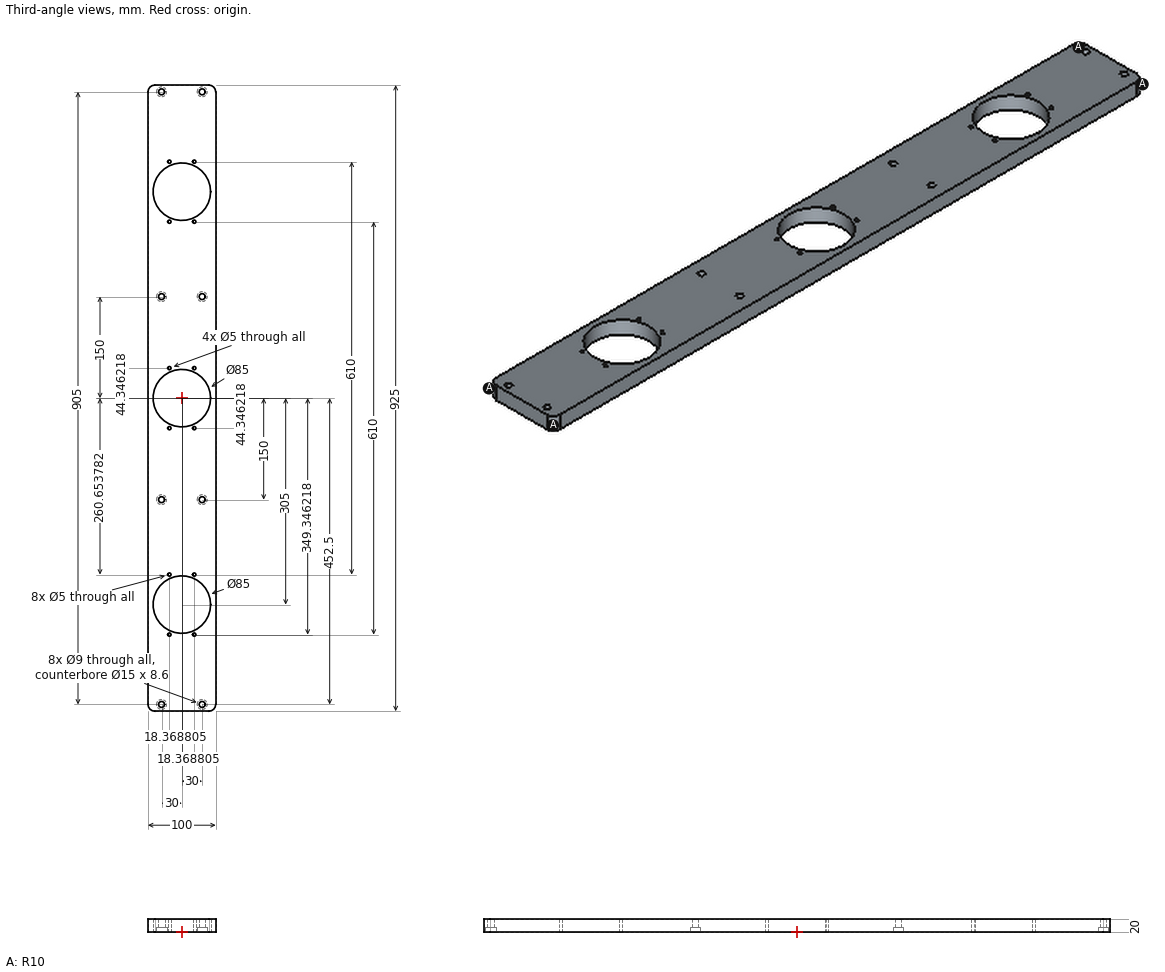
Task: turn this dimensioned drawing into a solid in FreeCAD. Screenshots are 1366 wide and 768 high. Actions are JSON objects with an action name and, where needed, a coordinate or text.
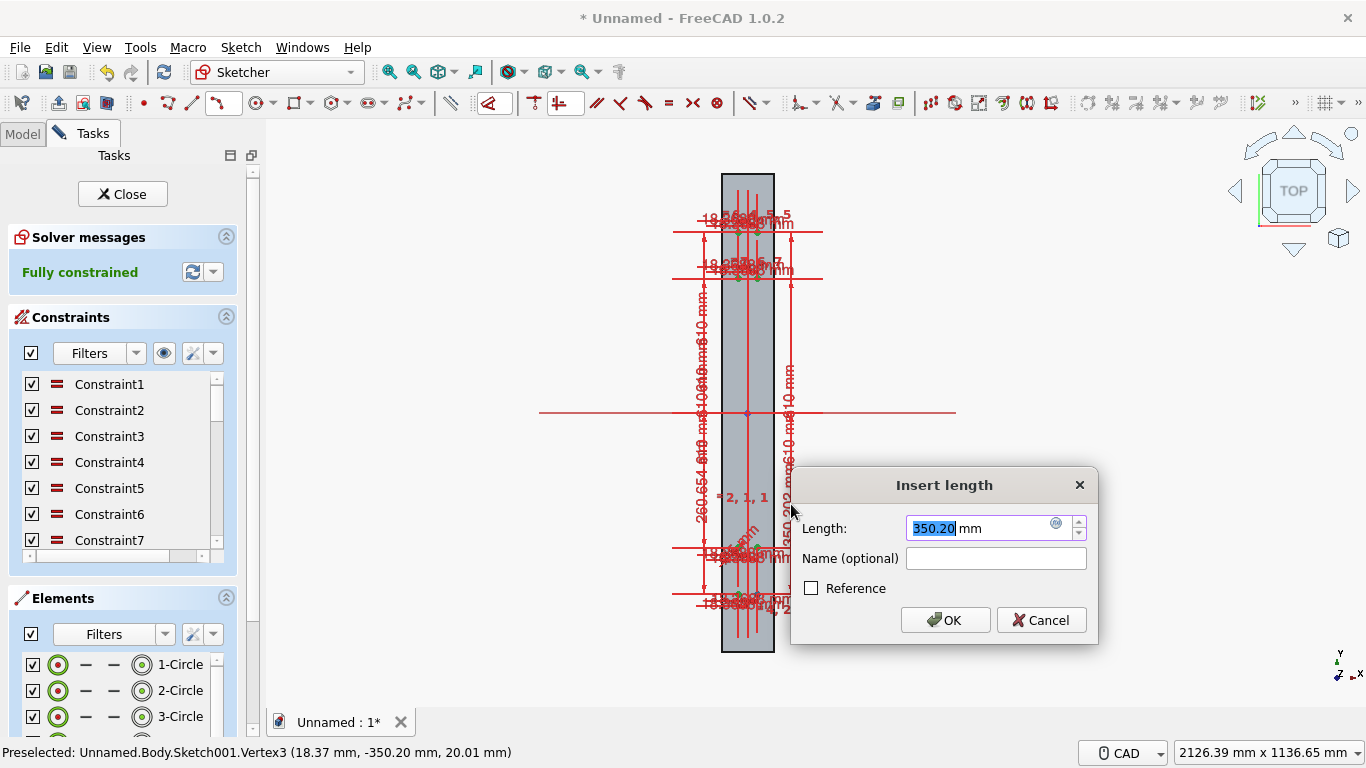
{"action": "type", "text": "349.346218"}
{"action": "key", "text": "Return"}
{"action": "key", "text": "Escape"}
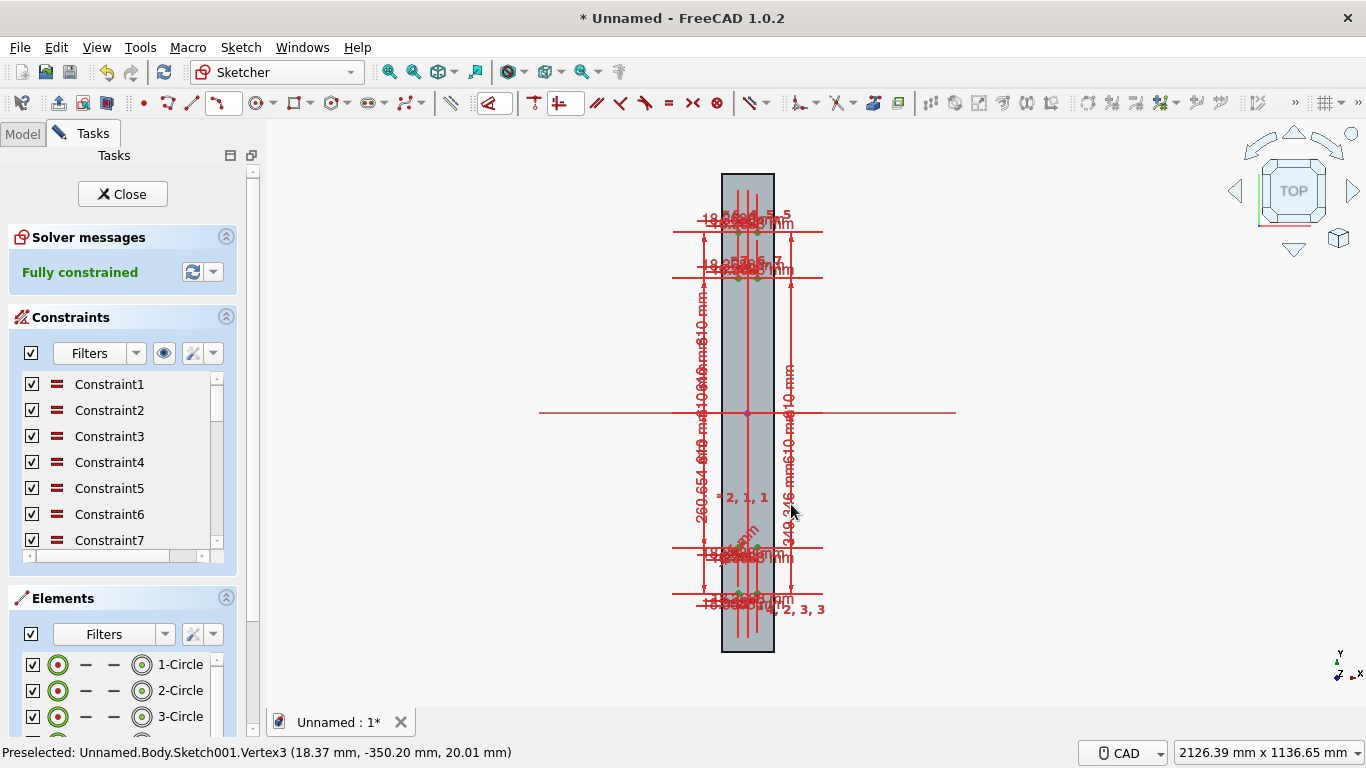
{"action": "left_click", "coordinate": [123, 194]}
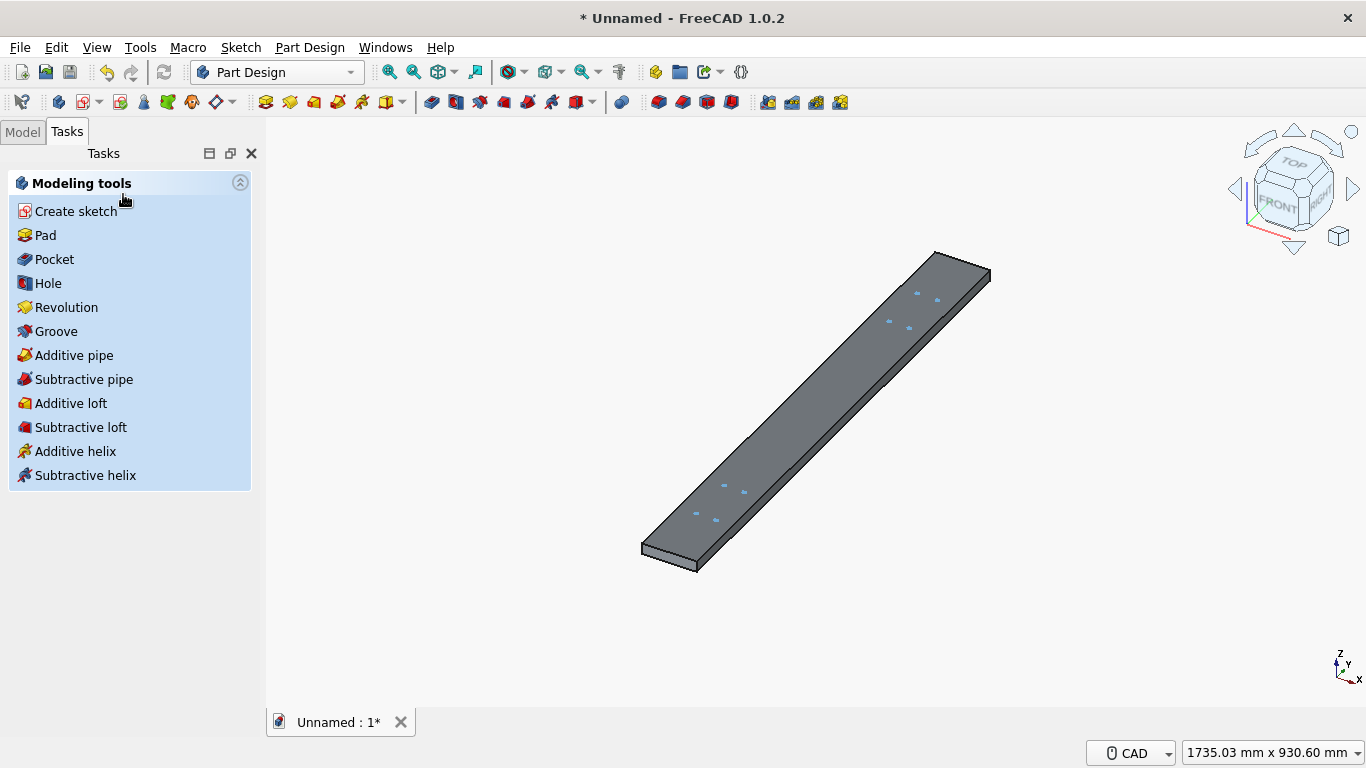
{"action": "left_click", "coordinate": [456, 102]}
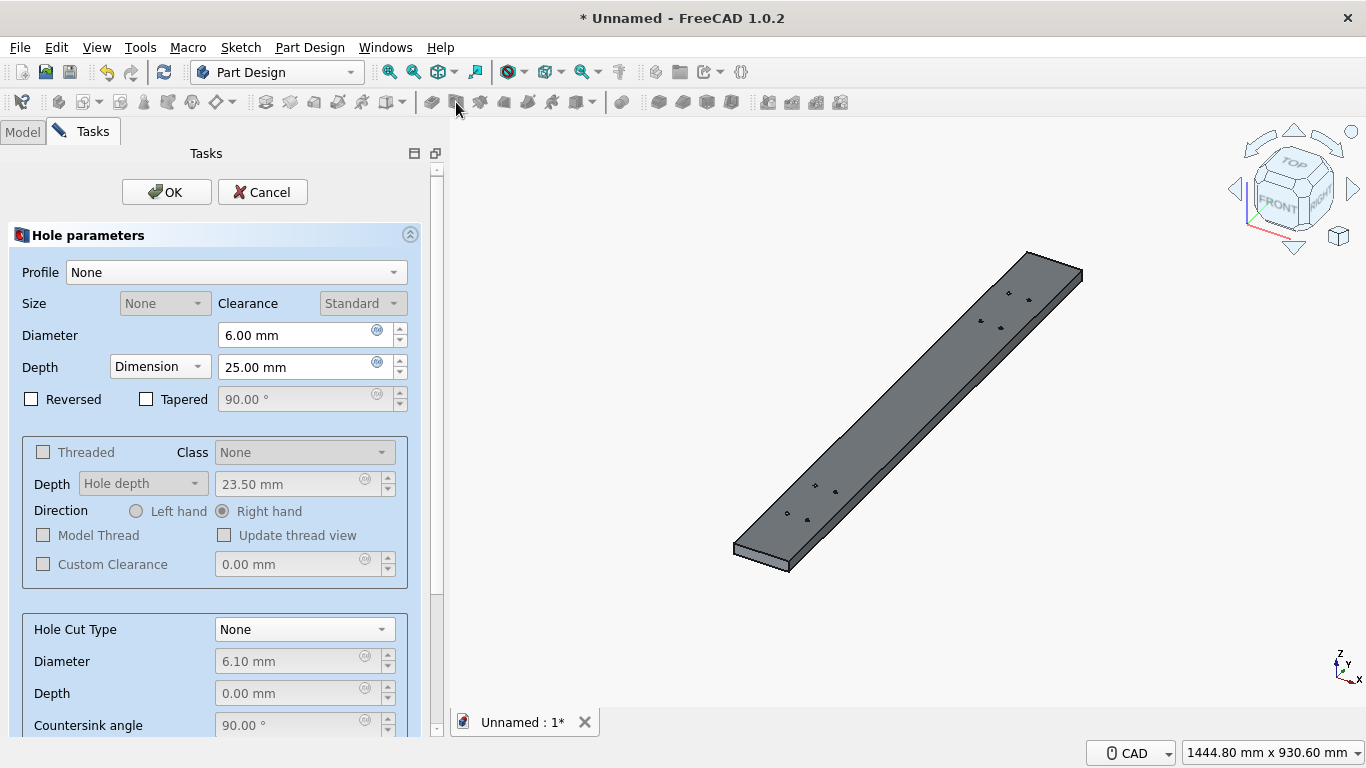
{"action": "triple_click", "coordinate": [305, 335]}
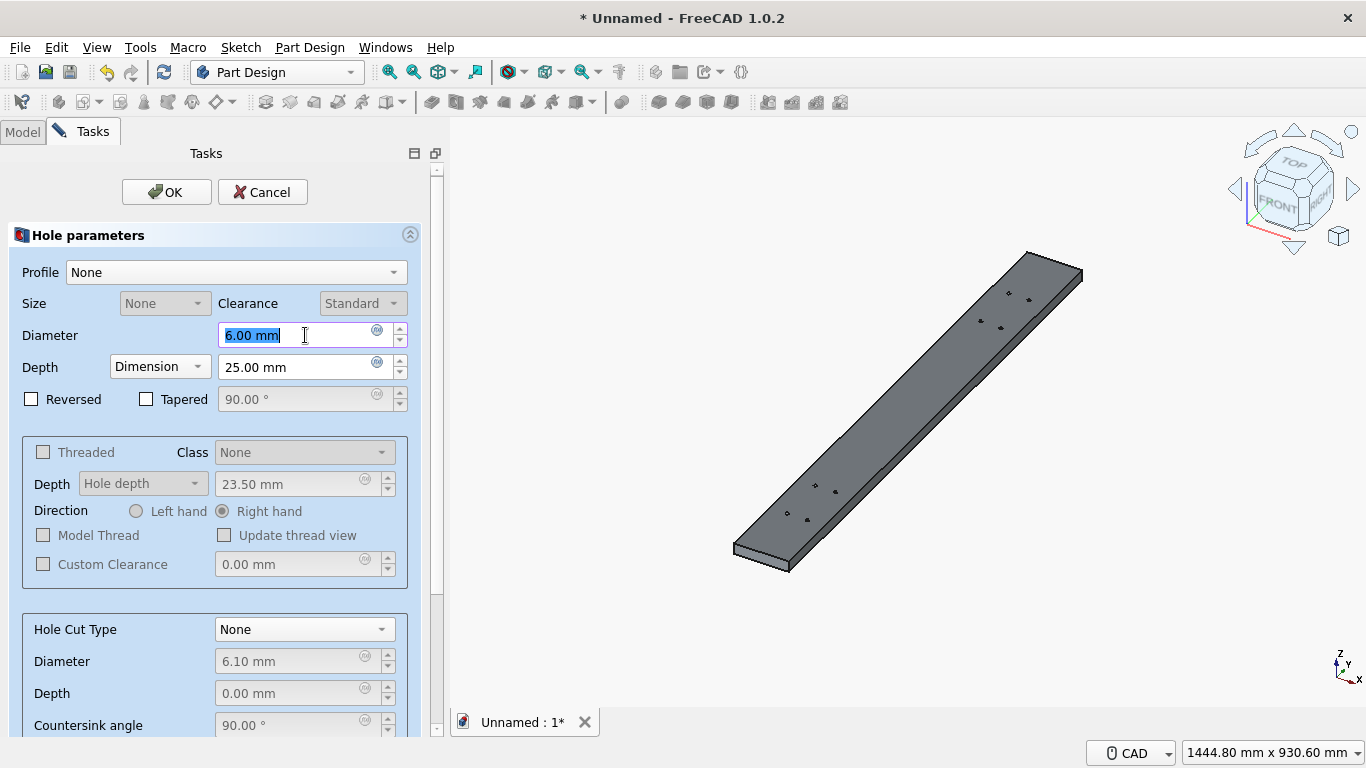
{"action": "type", "text": "5"}
{"action": "key", "text": "Tab"}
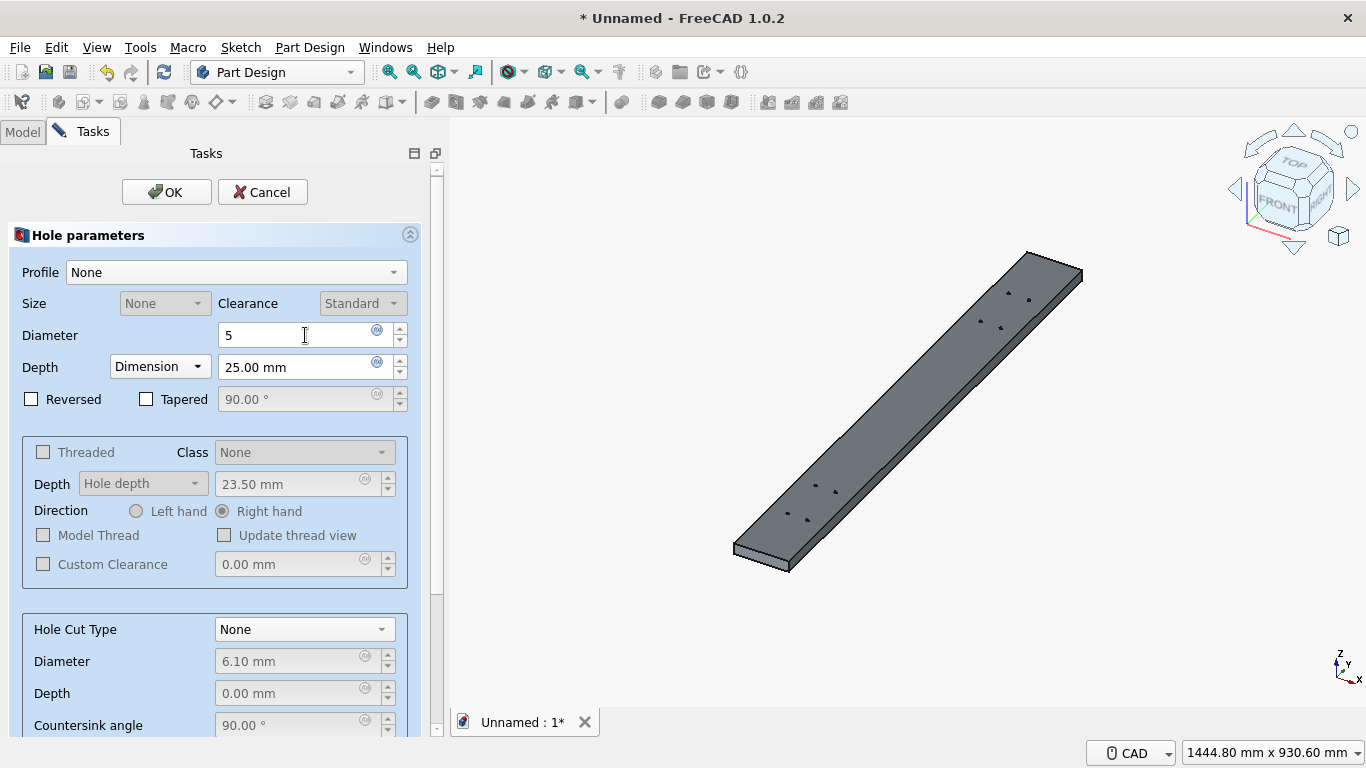
{"action": "left_click", "coordinate": [161, 366]}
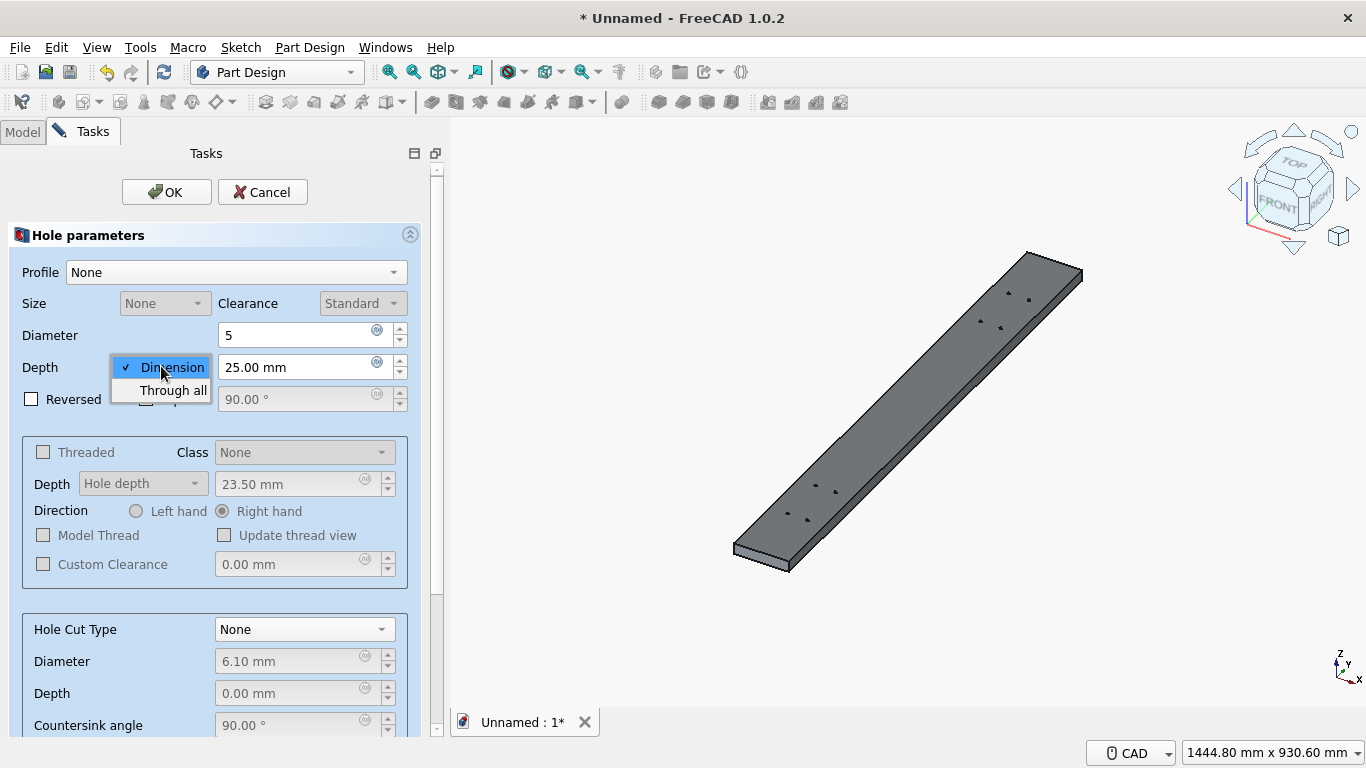
{"action": "left_click", "coordinate": [160, 390]}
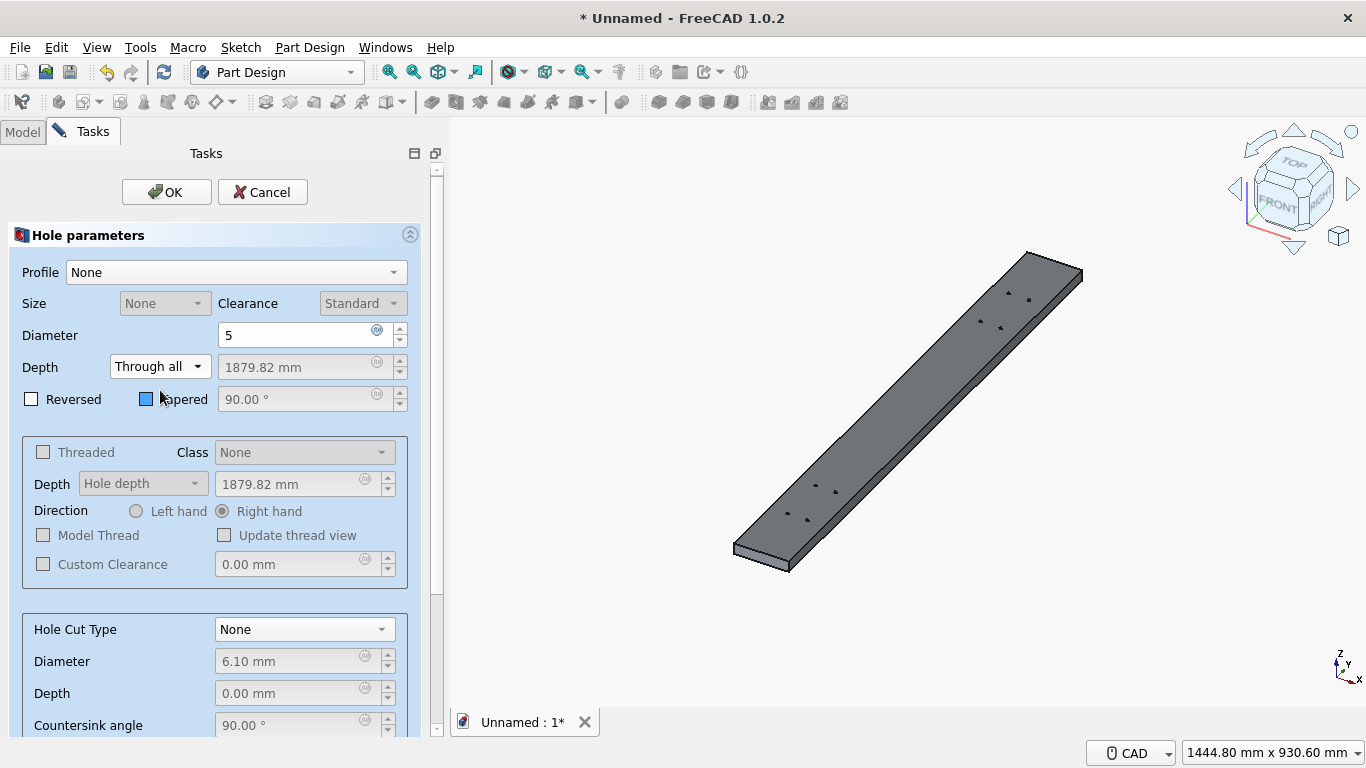
{"action": "left_click", "coordinate": [167, 192]}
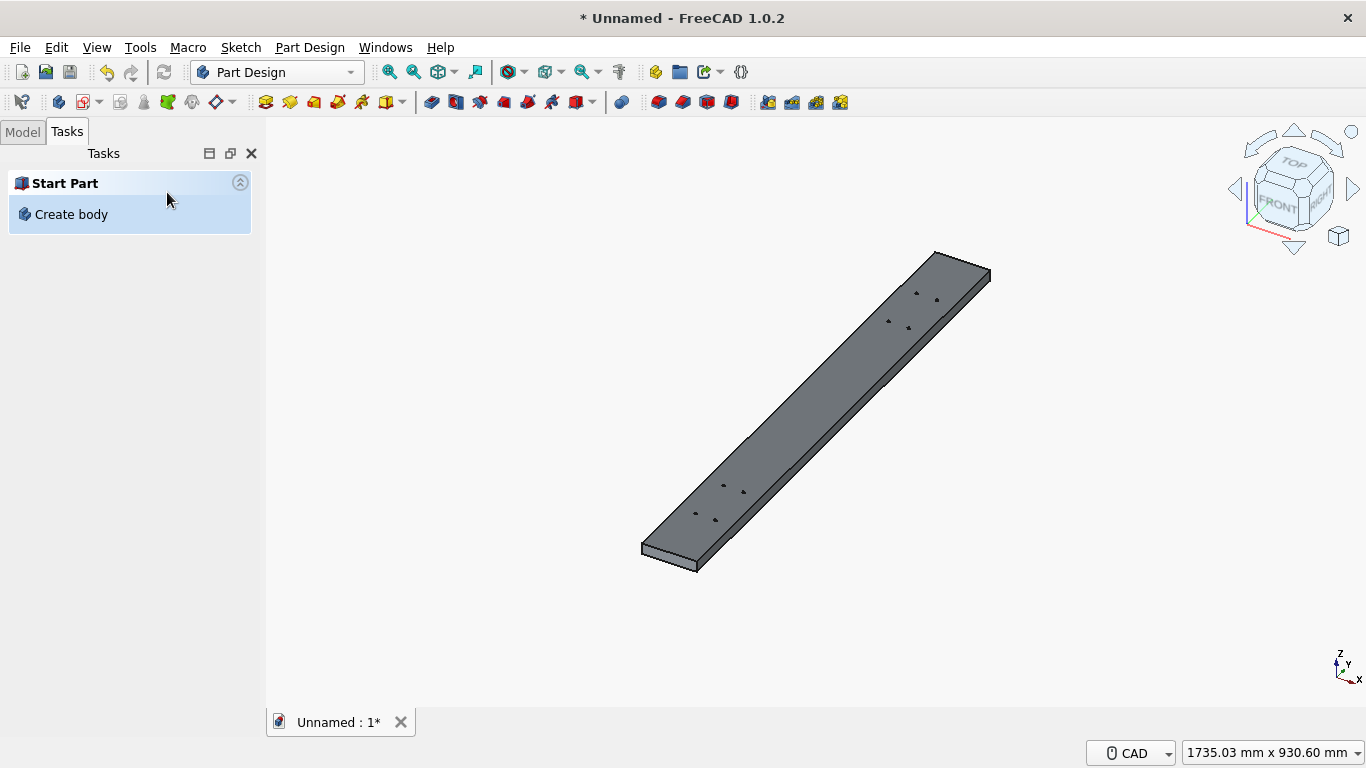
{"action": "left_click", "coordinate": [858, 364]}